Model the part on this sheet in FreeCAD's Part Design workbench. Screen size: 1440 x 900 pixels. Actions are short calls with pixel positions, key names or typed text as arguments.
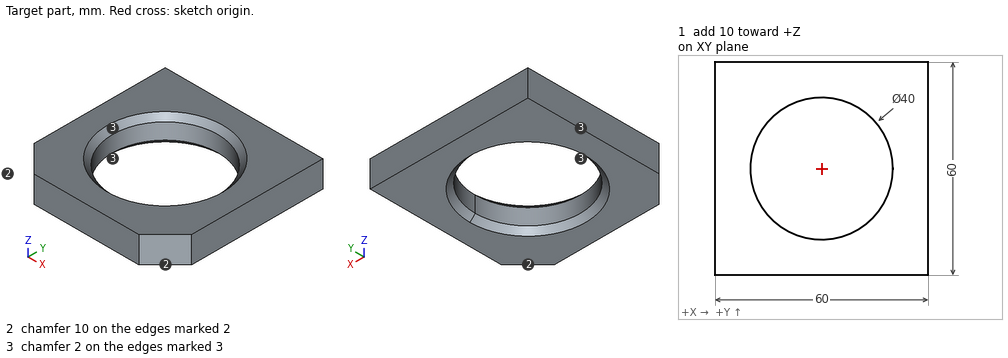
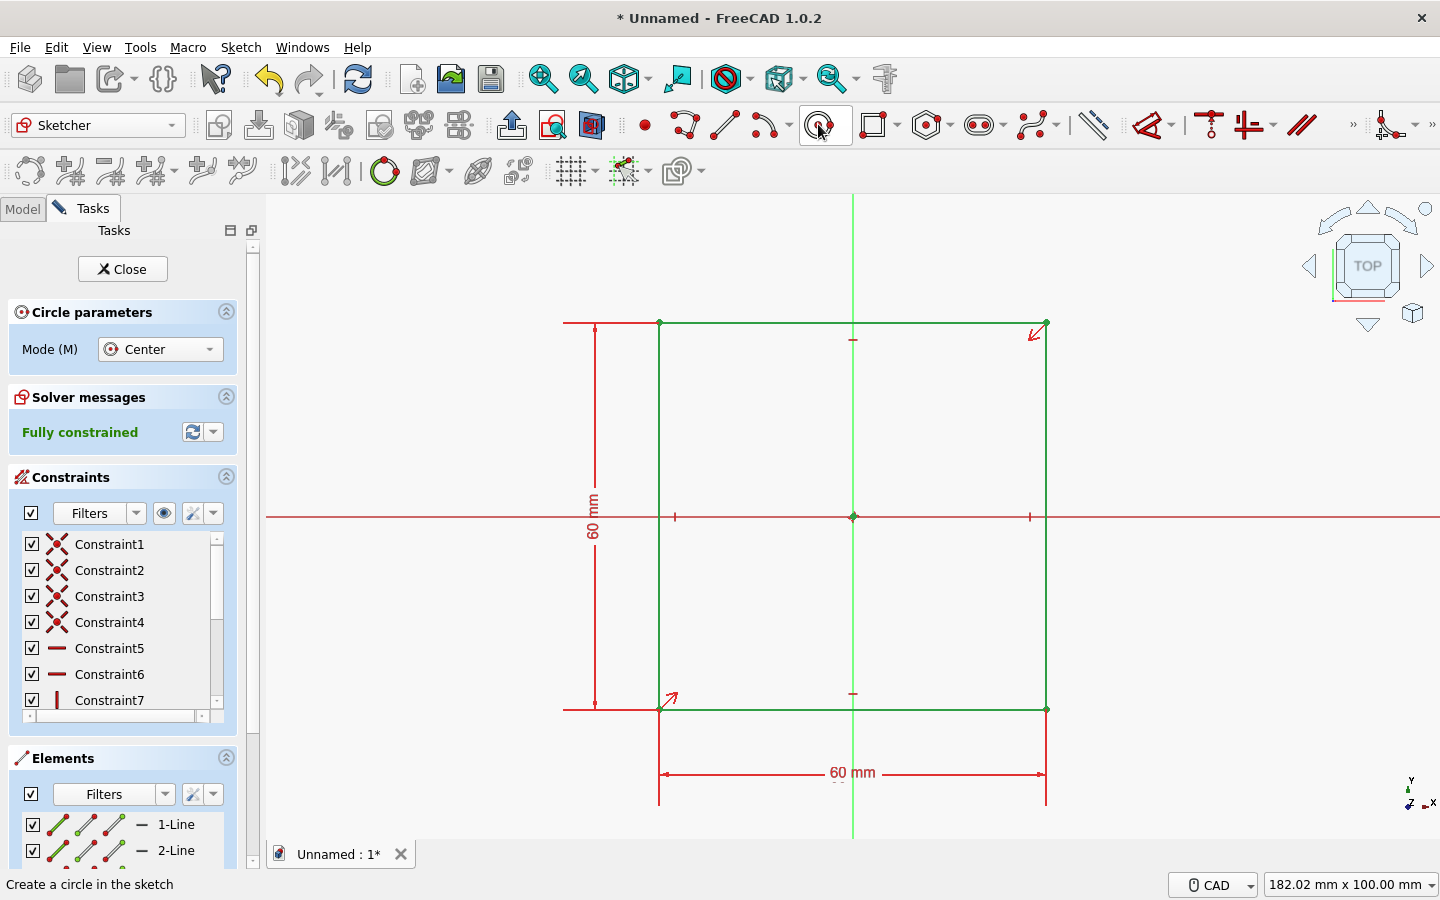
click(853, 516)
move(944, 425)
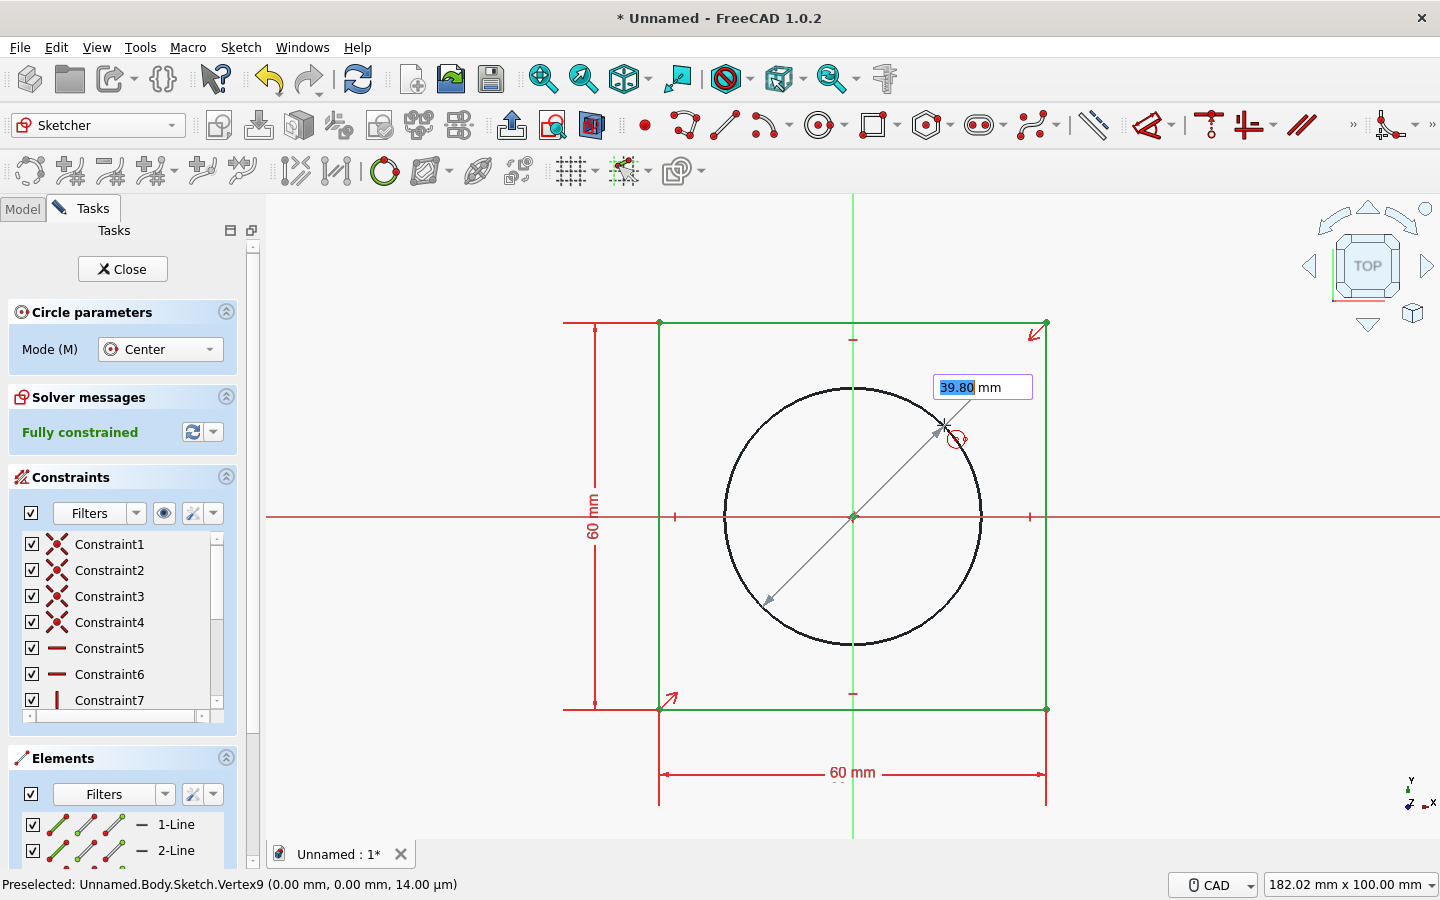
text(40)
key(Return)
key(Escape)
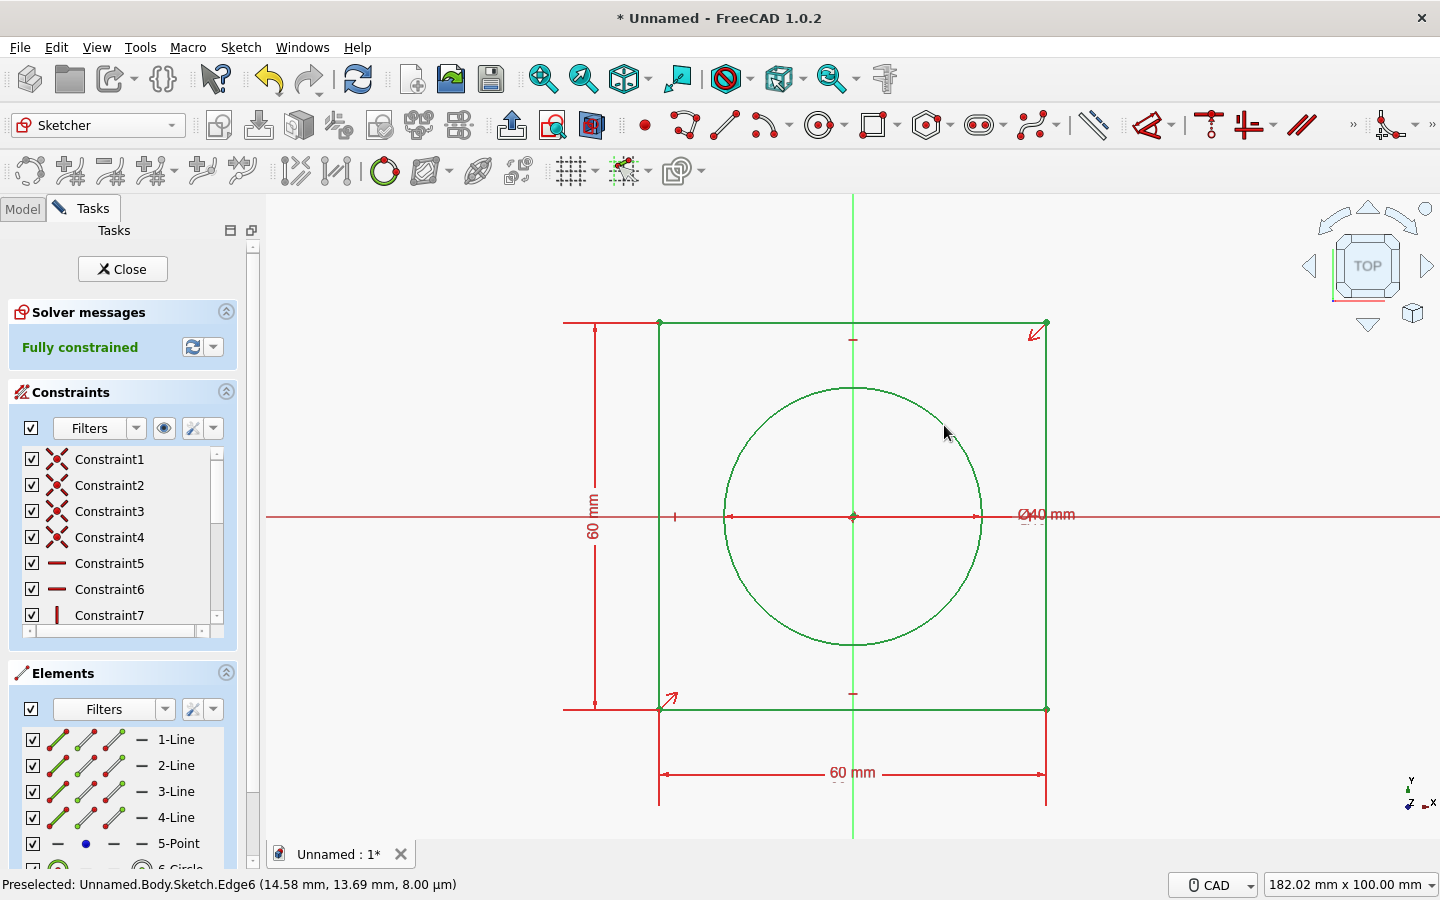
click(123, 269)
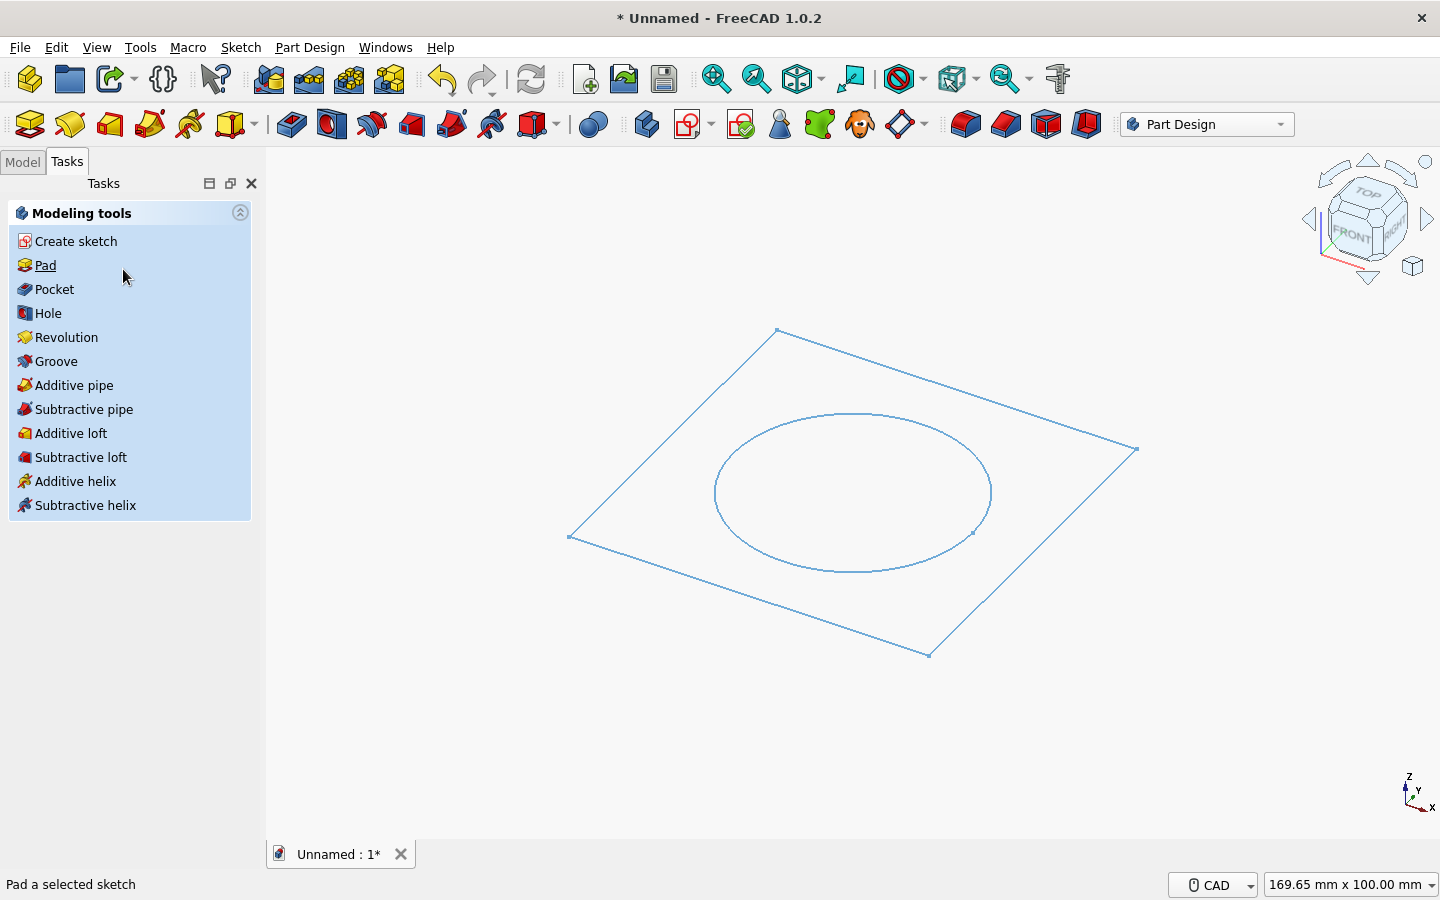
click(30, 124)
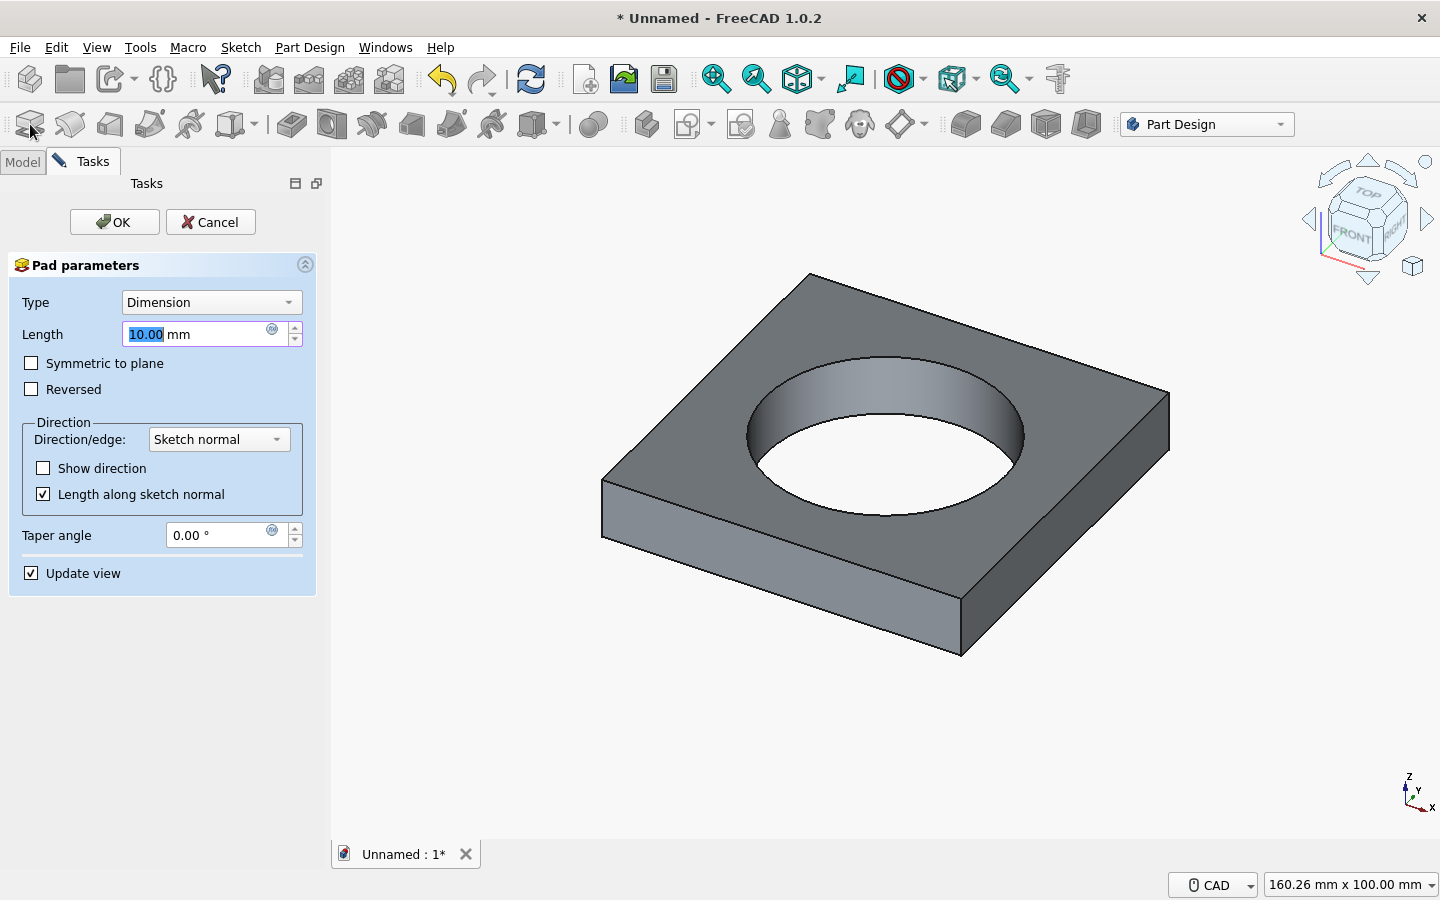
text(10)
key(Tab)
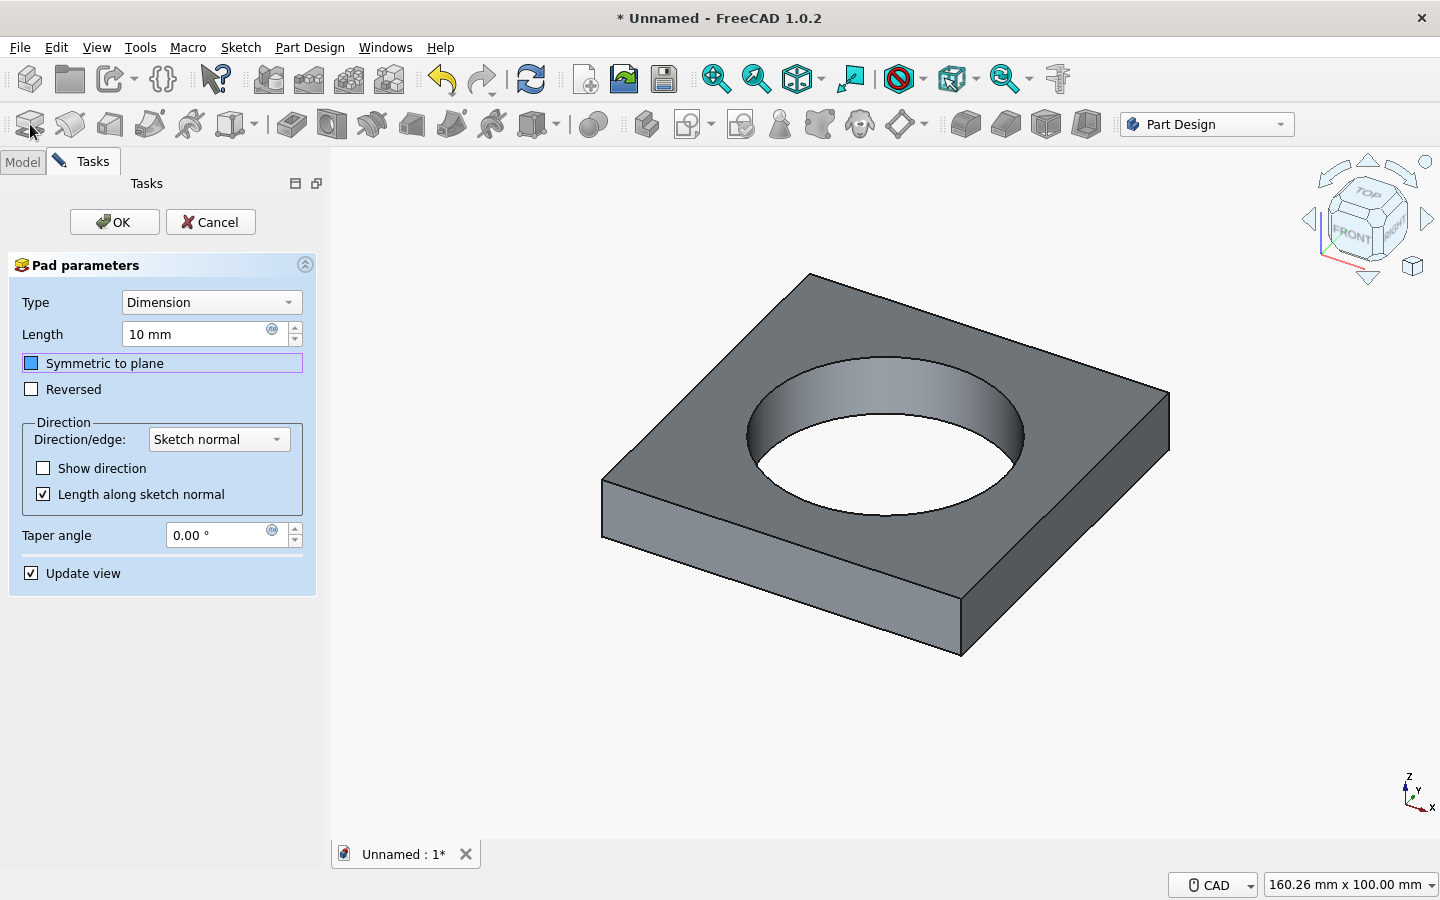
click(115, 222)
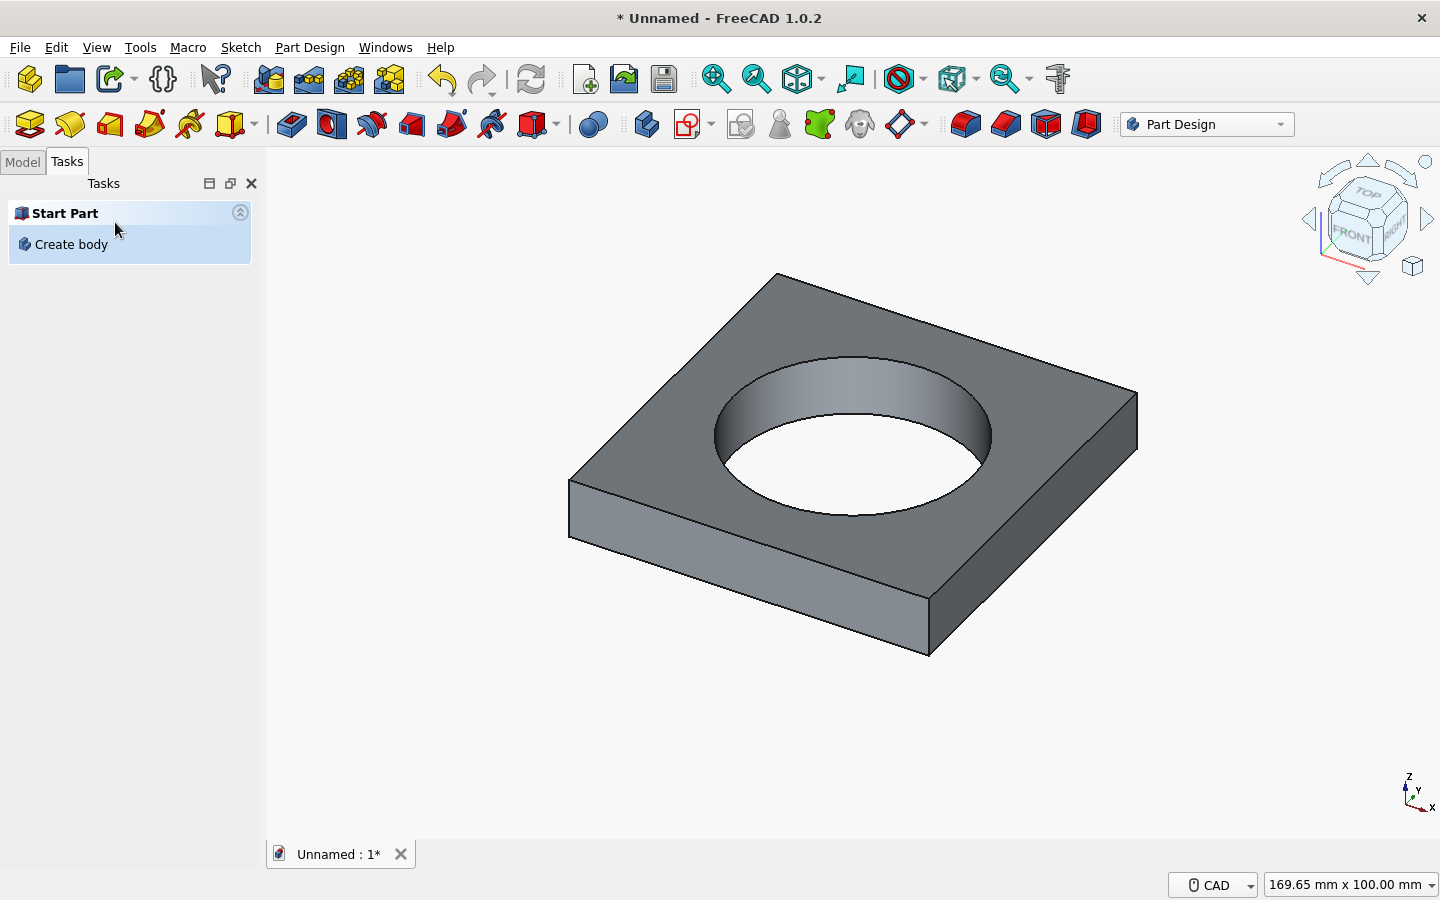
click(929, 626)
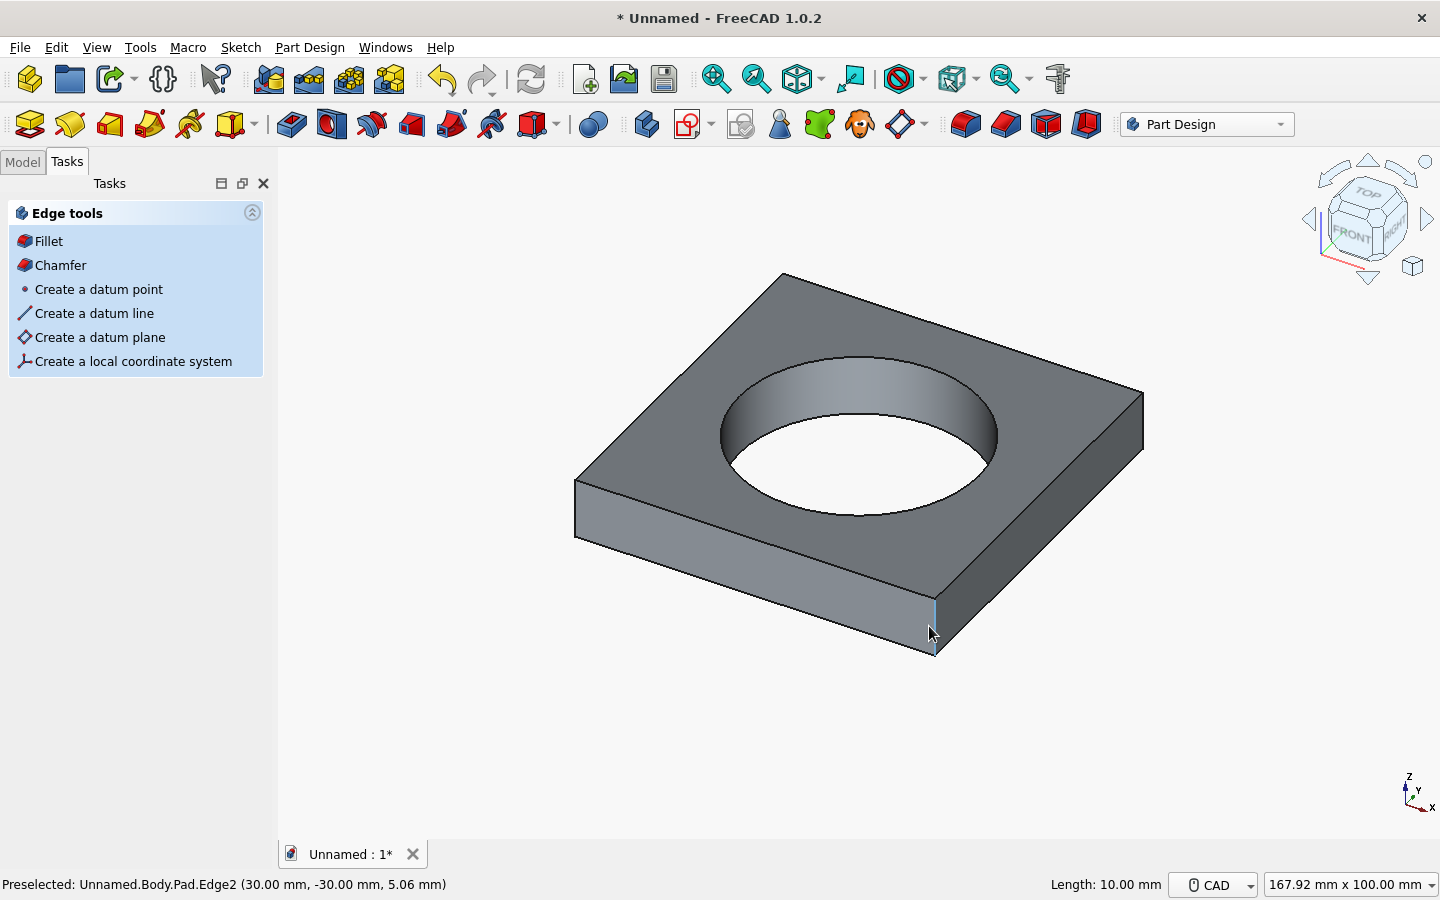
key(0)